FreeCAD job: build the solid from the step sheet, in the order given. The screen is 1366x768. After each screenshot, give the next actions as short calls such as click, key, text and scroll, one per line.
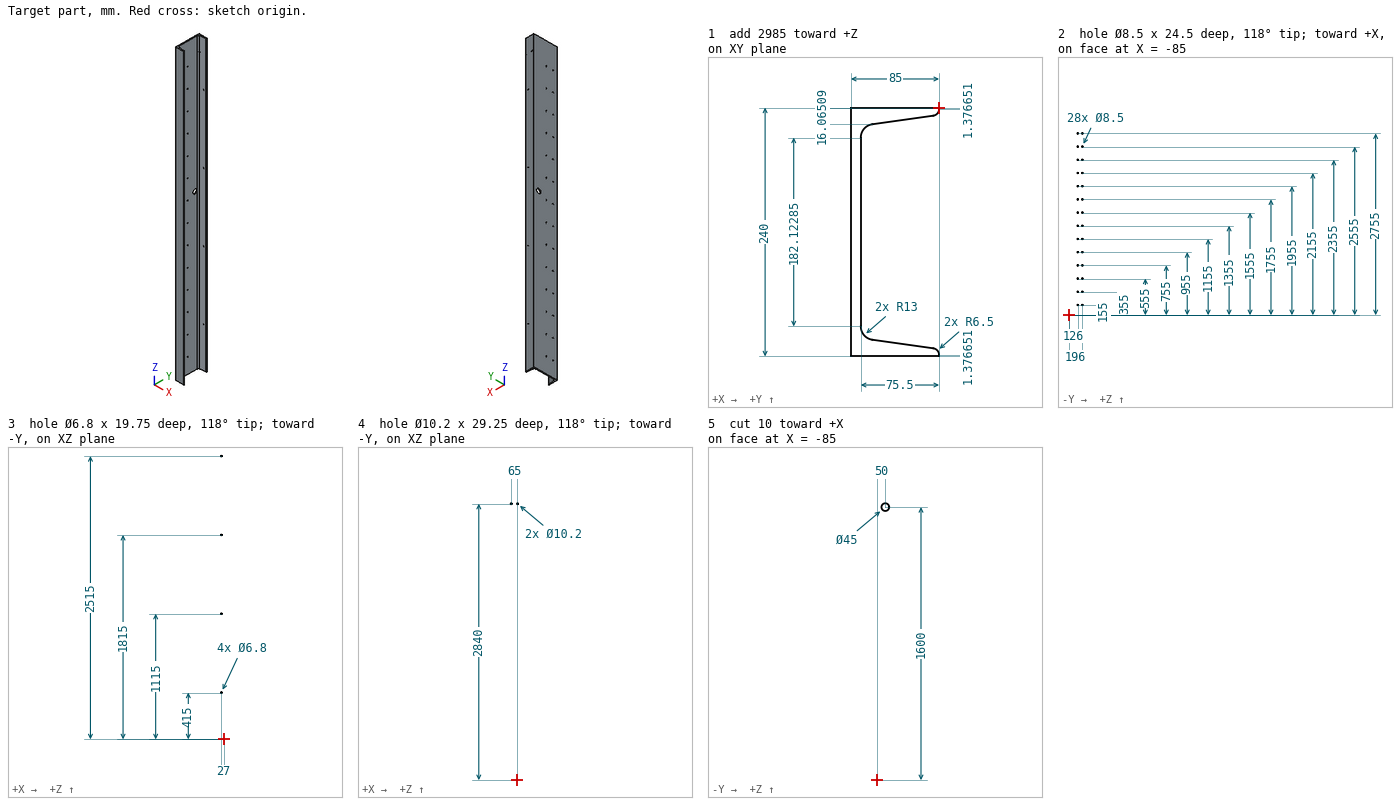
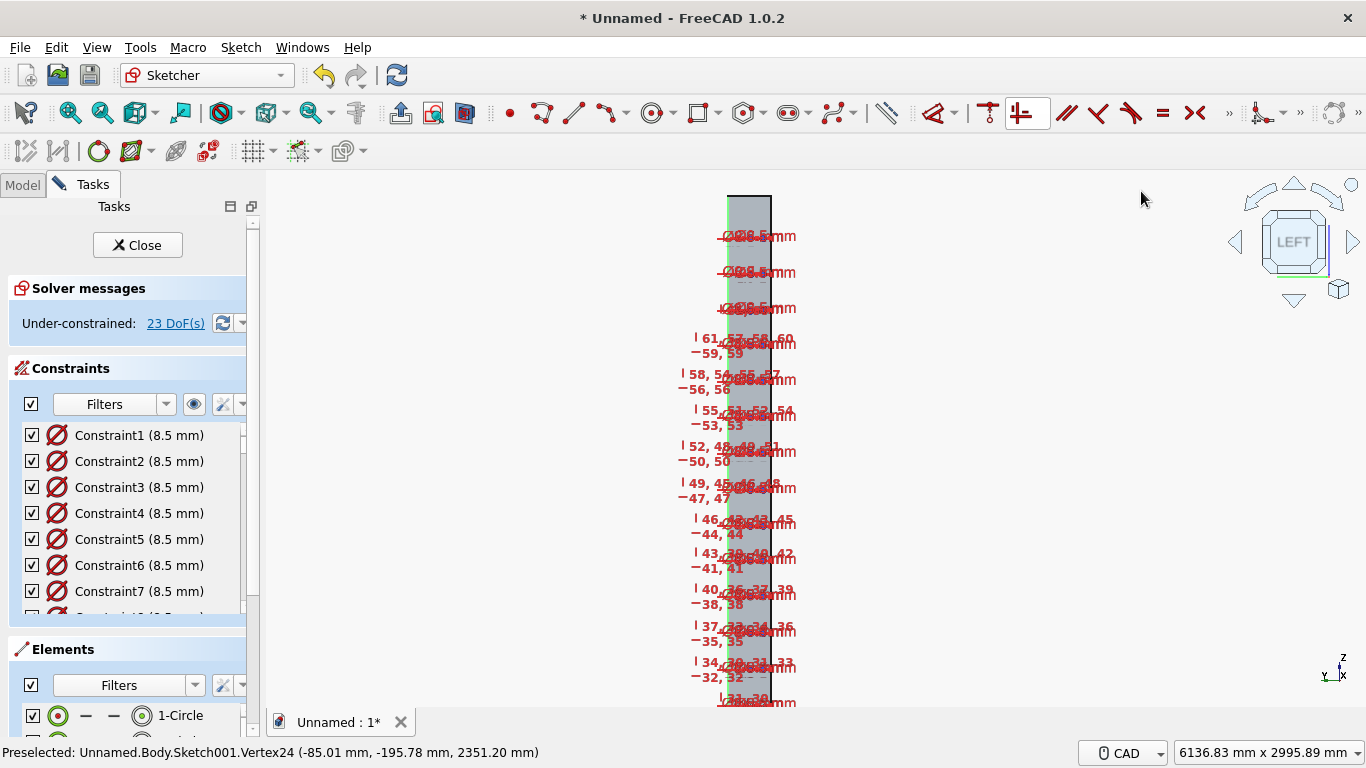
scroll(750, 311, up, 4)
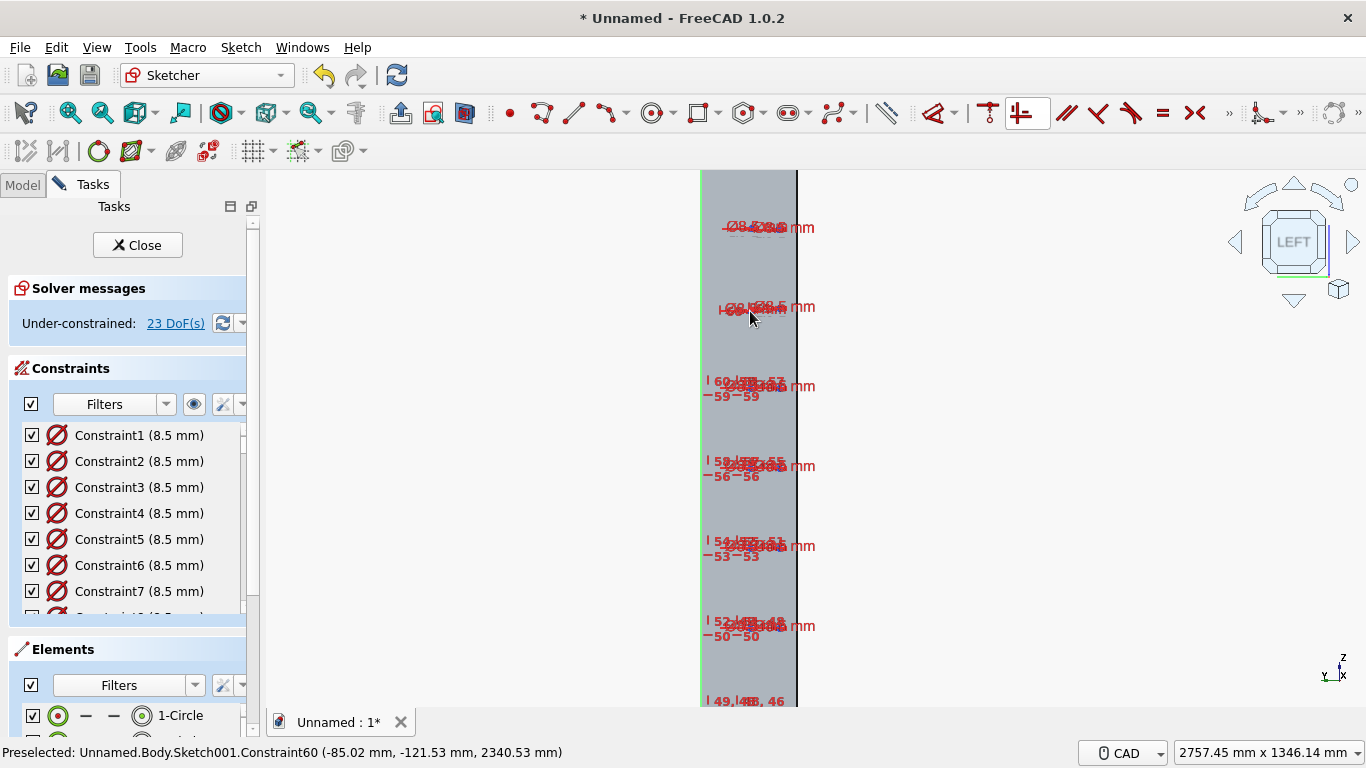
scroll(750, 311, up, 4)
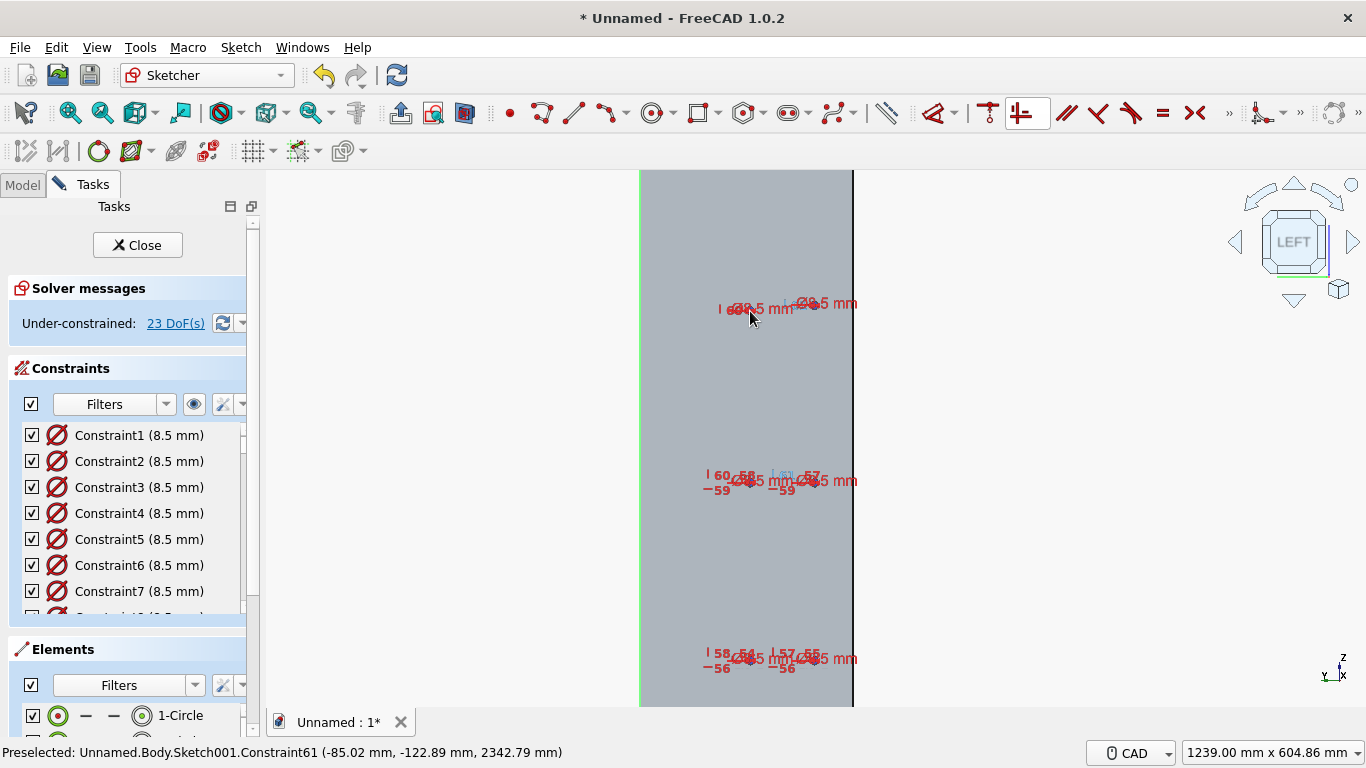
click(750, 311)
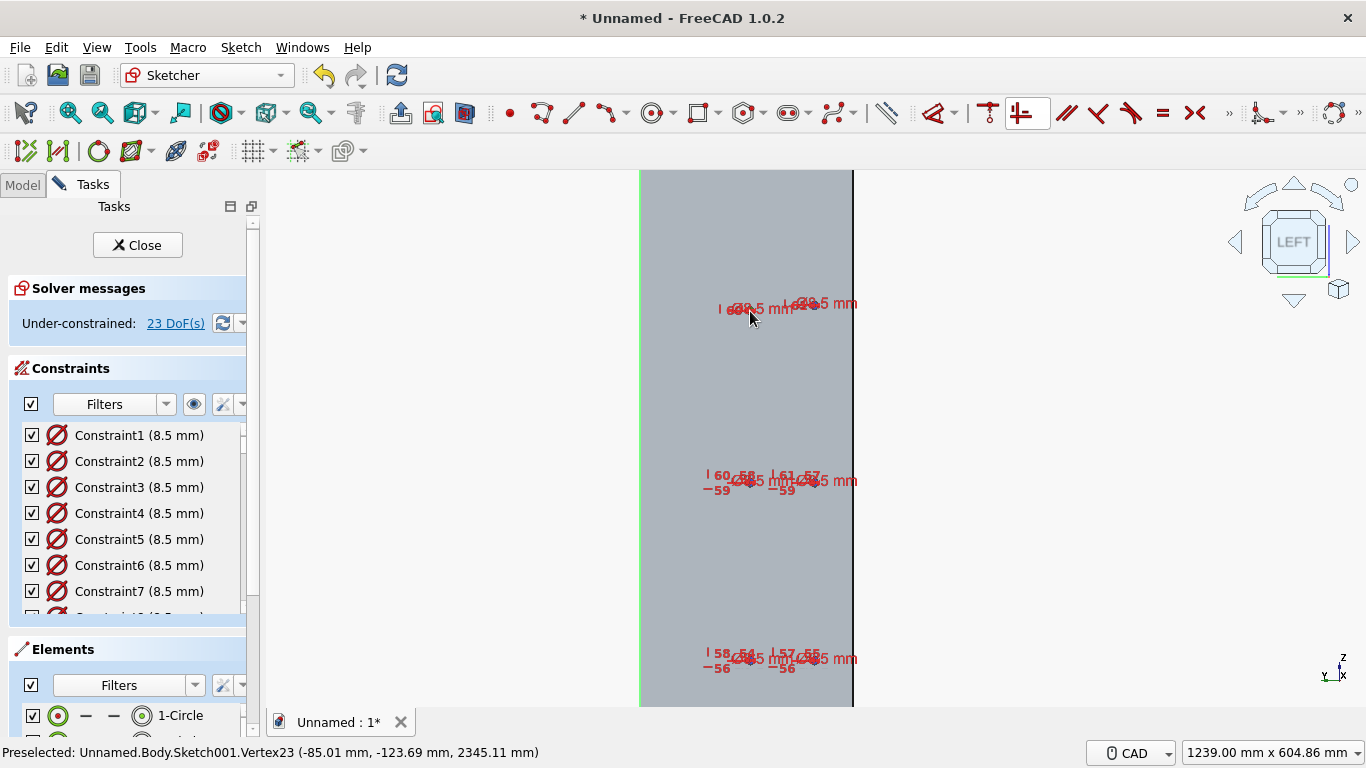
scroll(750, 324, down, 10)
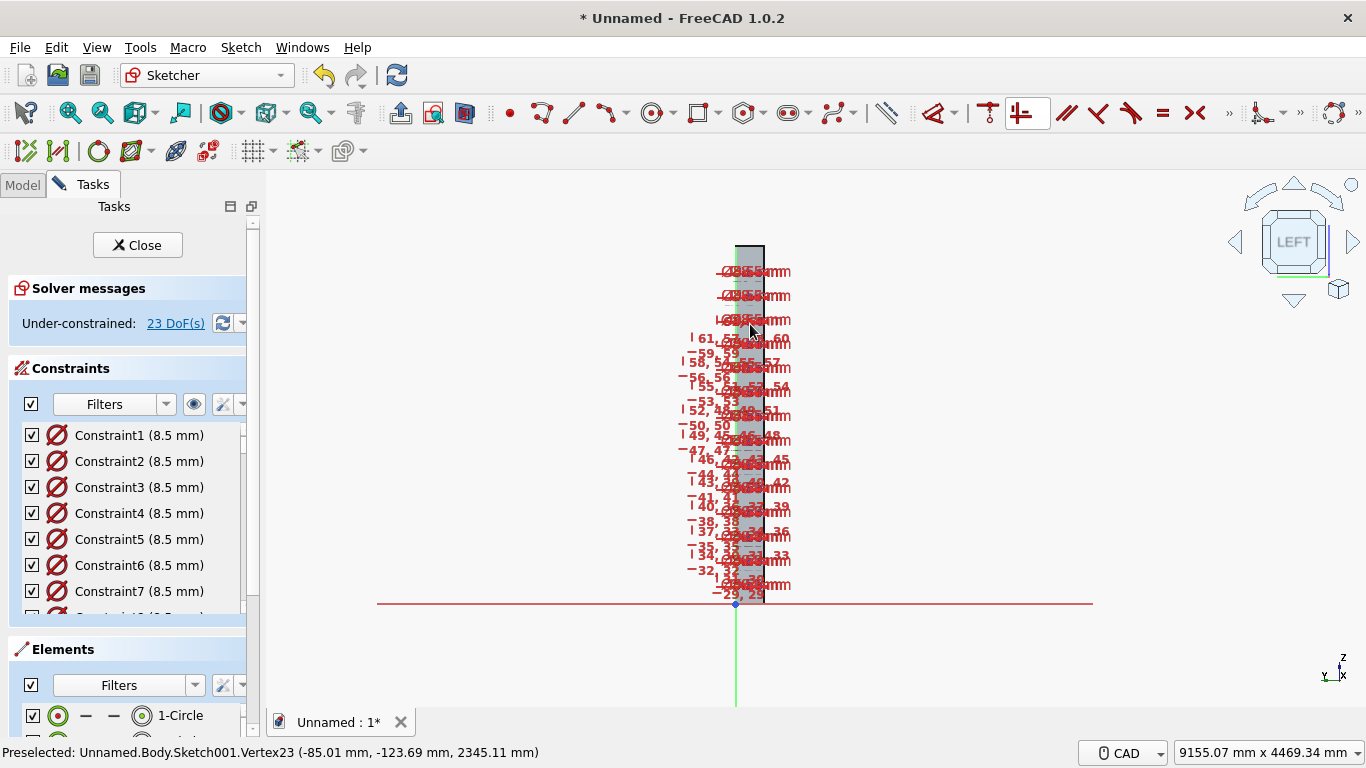
scroll(759, 322, up, 2)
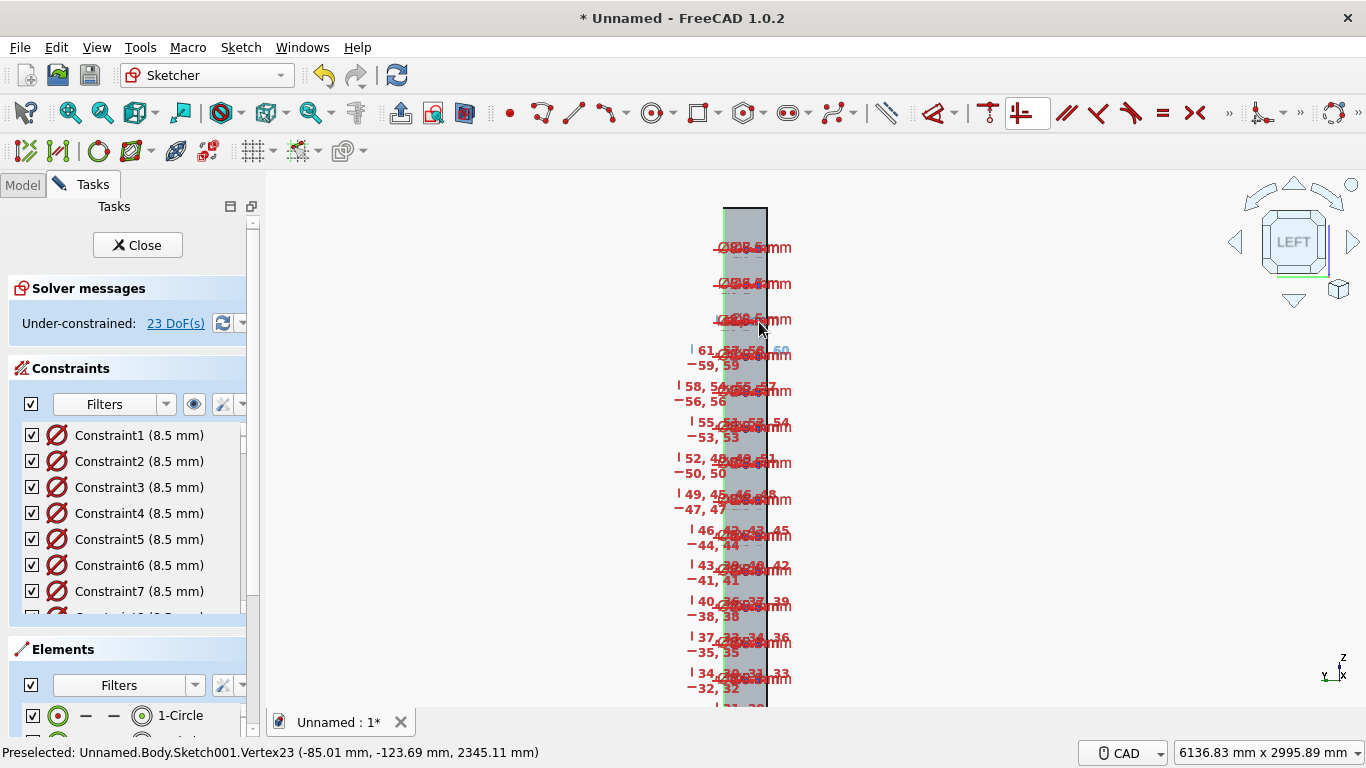
scroll(759, 321, up, 4)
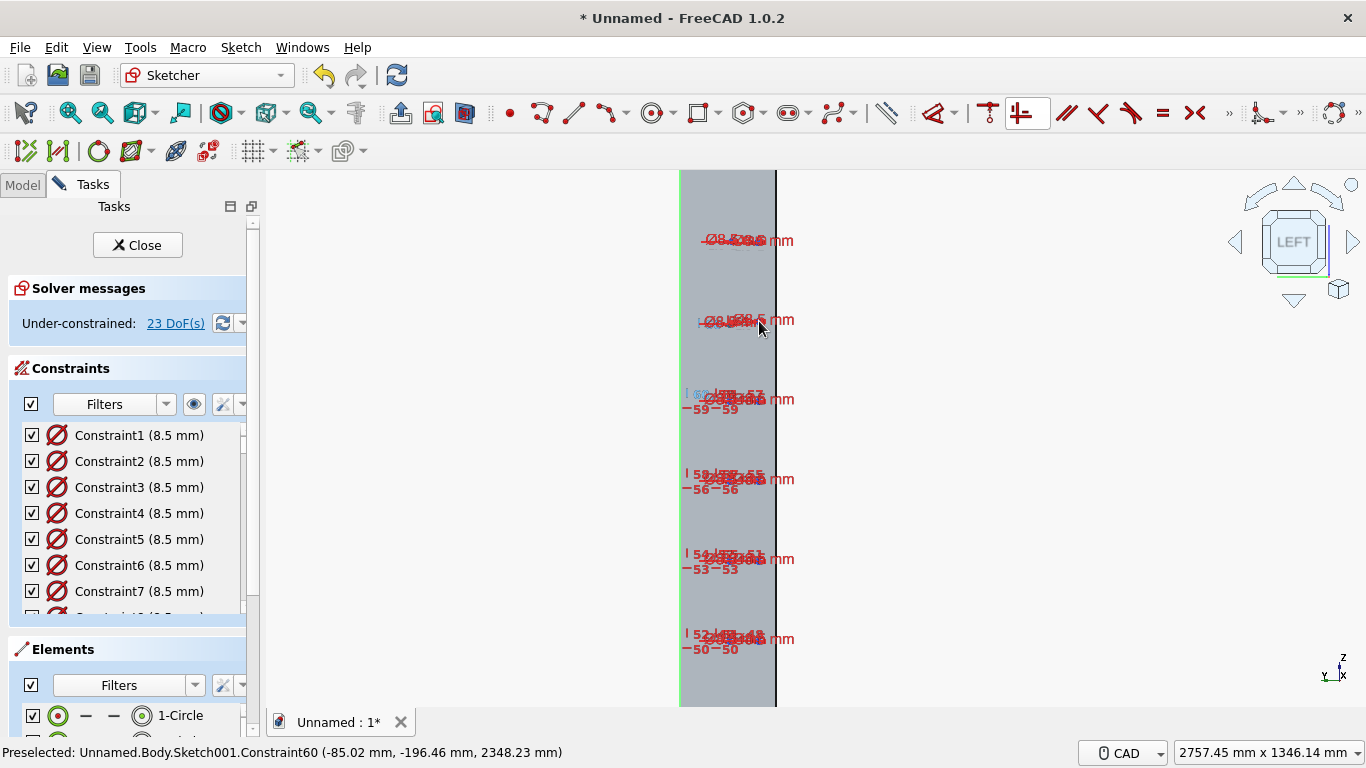
click(758, 322)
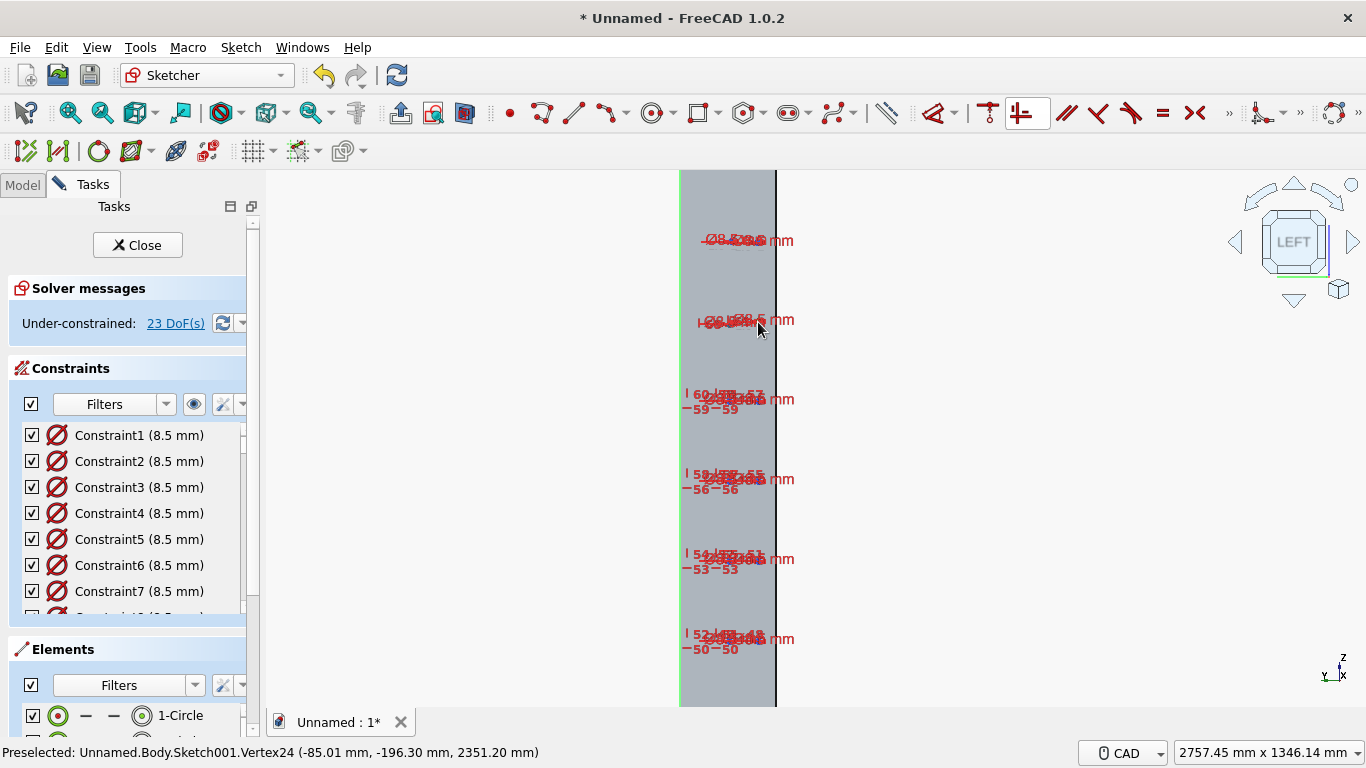
click(1044, 114)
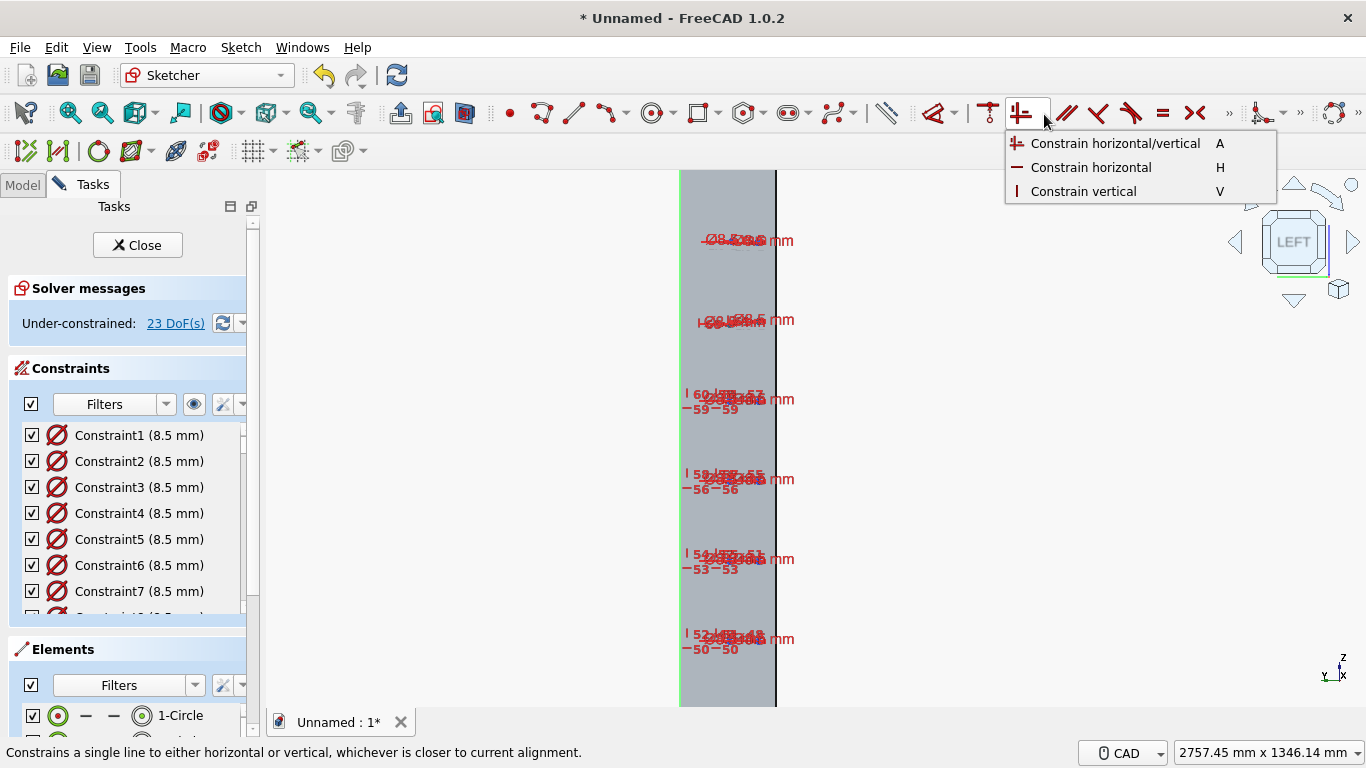
click(1141, 167)